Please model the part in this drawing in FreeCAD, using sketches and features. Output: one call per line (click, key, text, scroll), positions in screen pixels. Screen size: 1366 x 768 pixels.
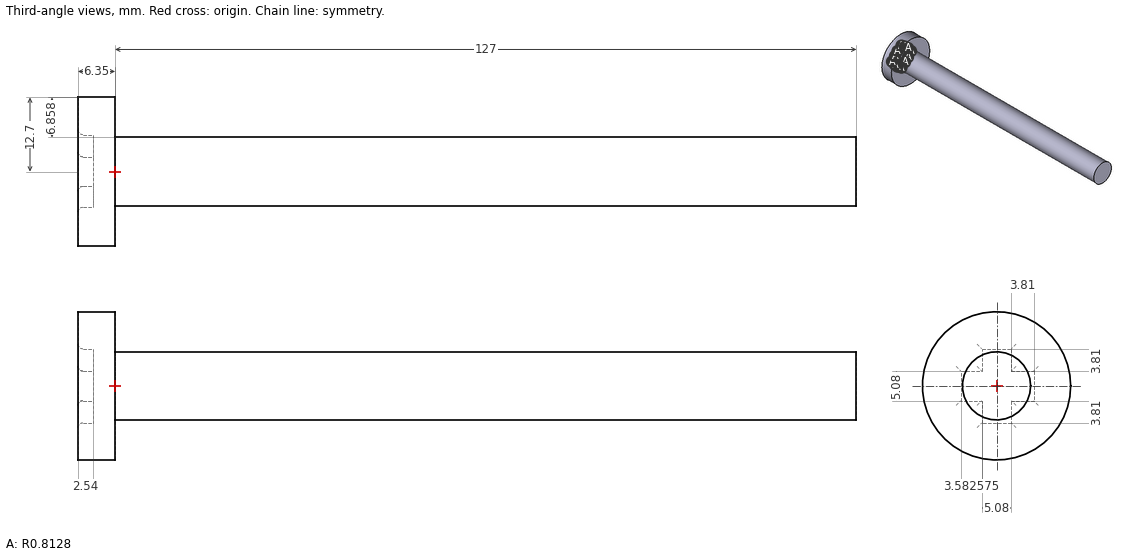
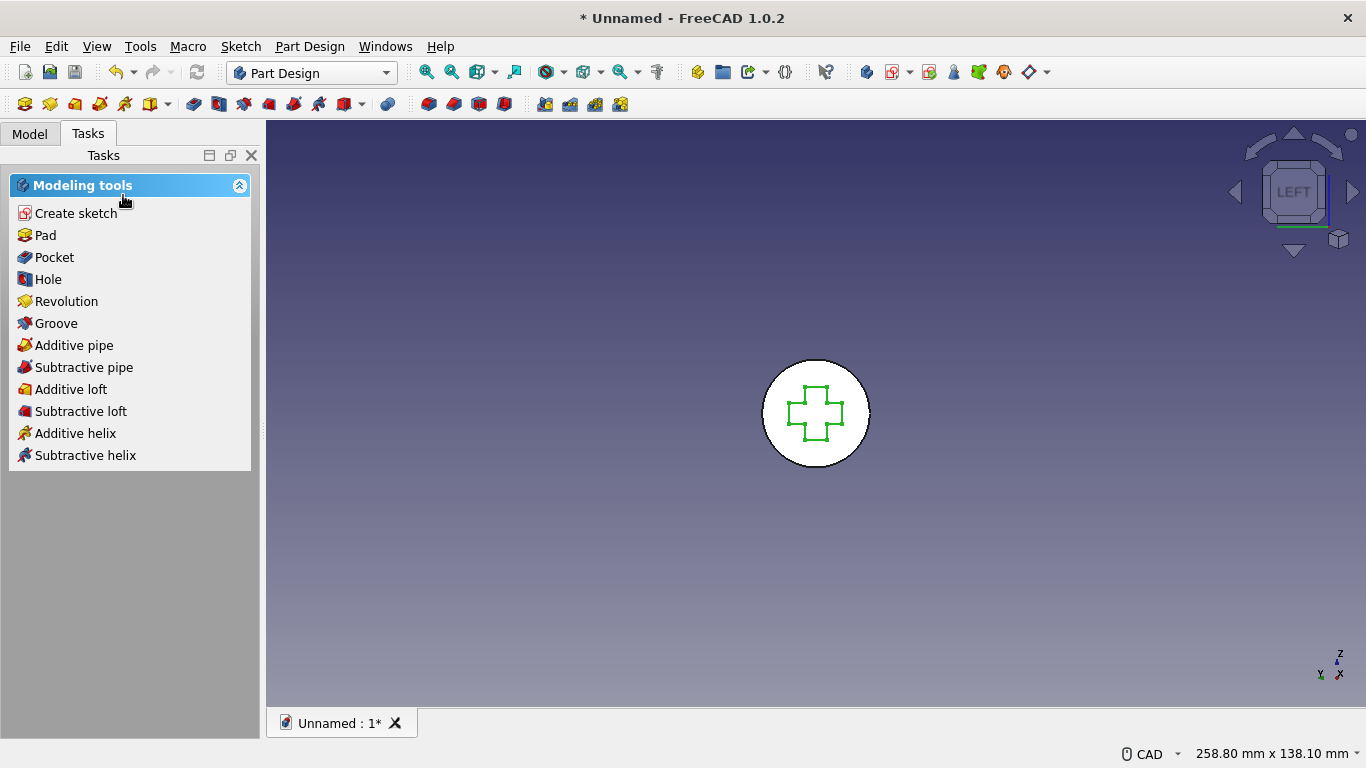
click(194, 104)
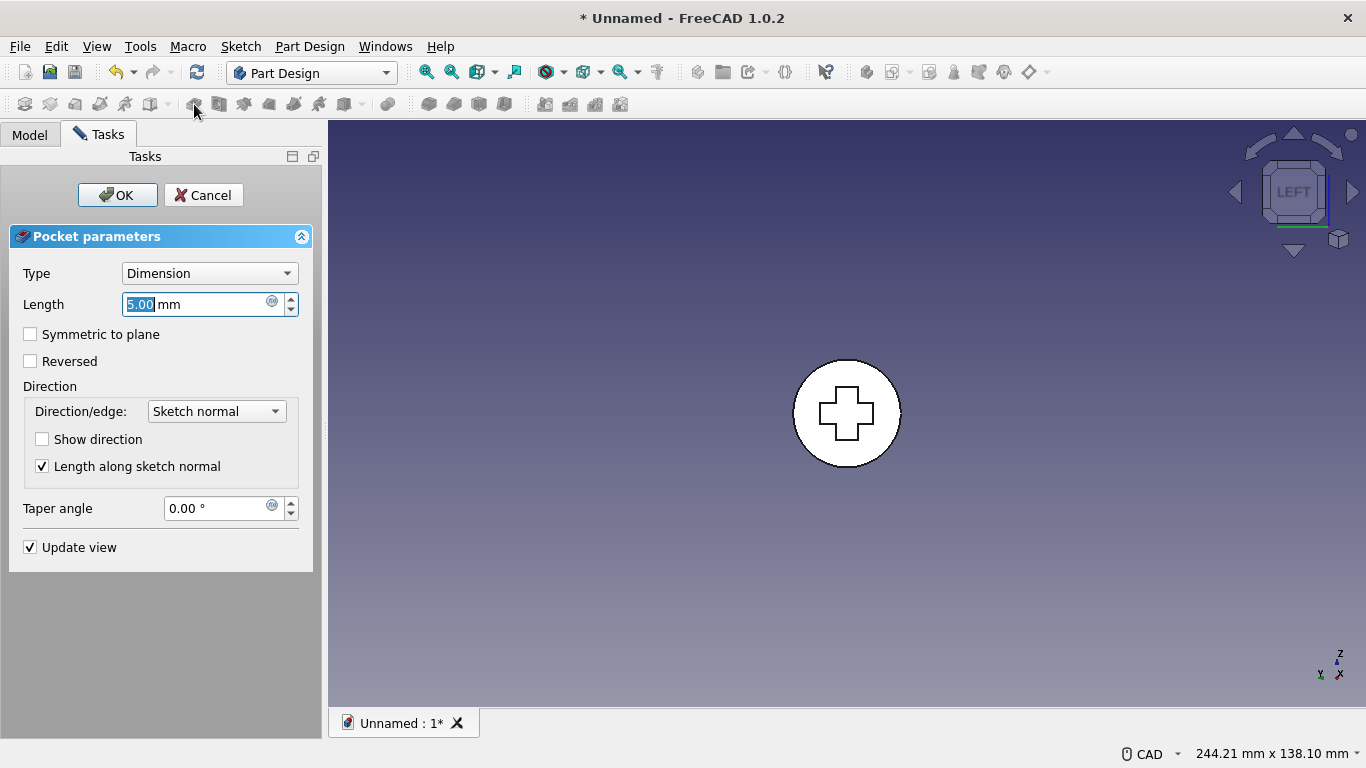
text(2.54)
key(Tab)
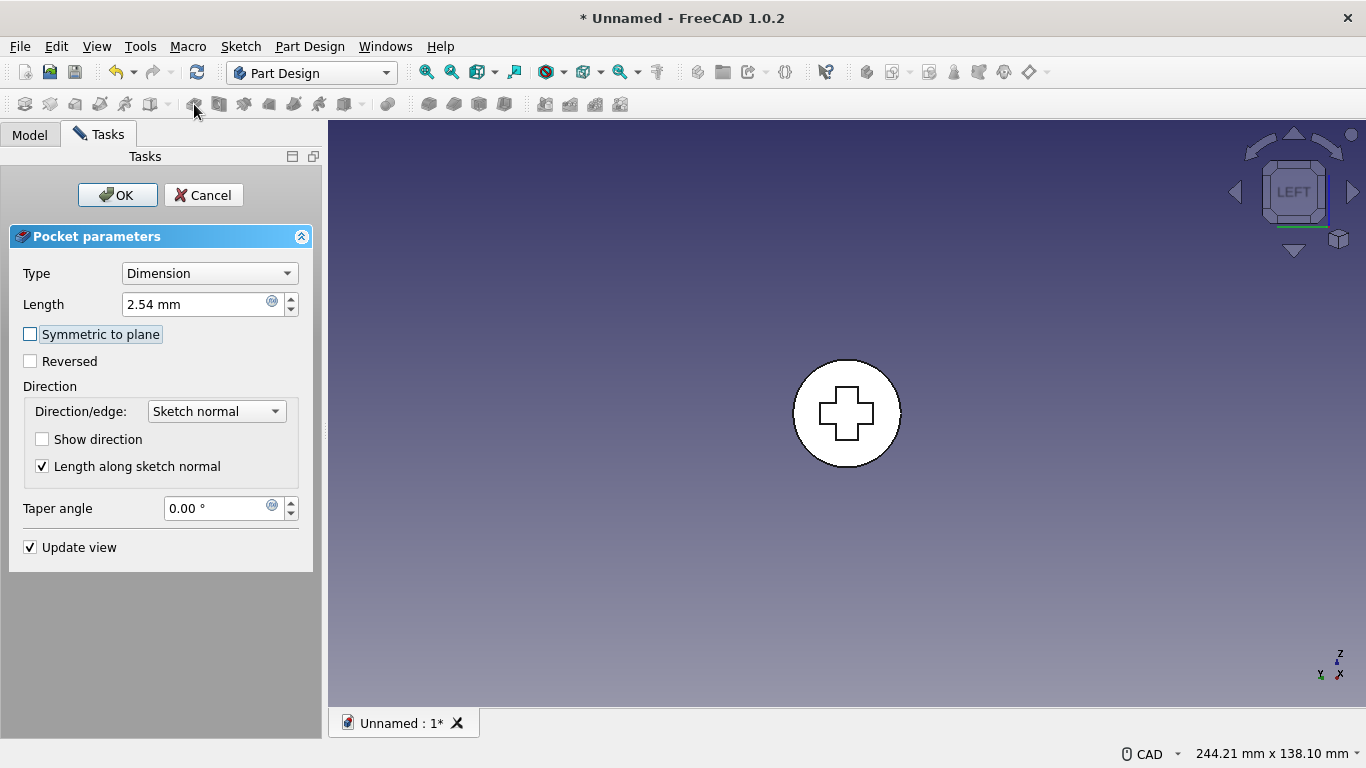
click(118, 195)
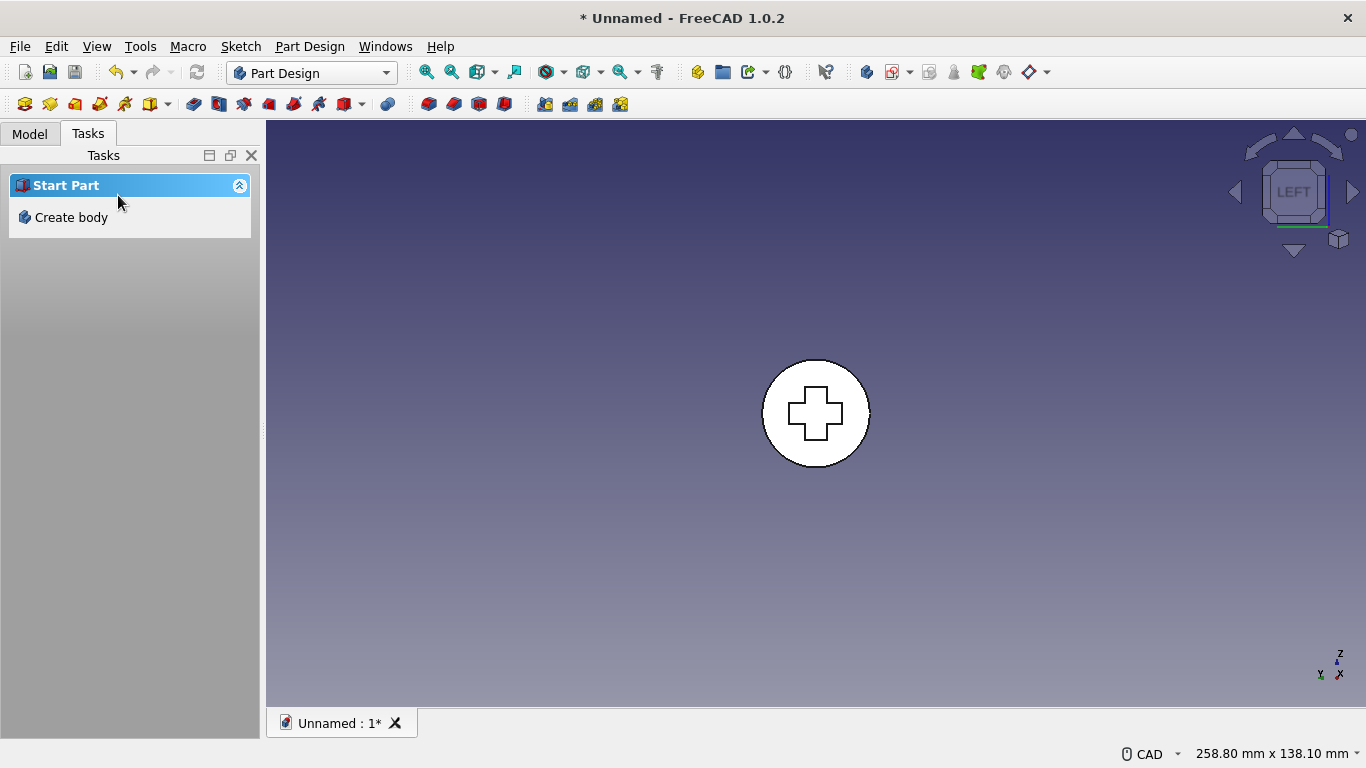
click(427, 72)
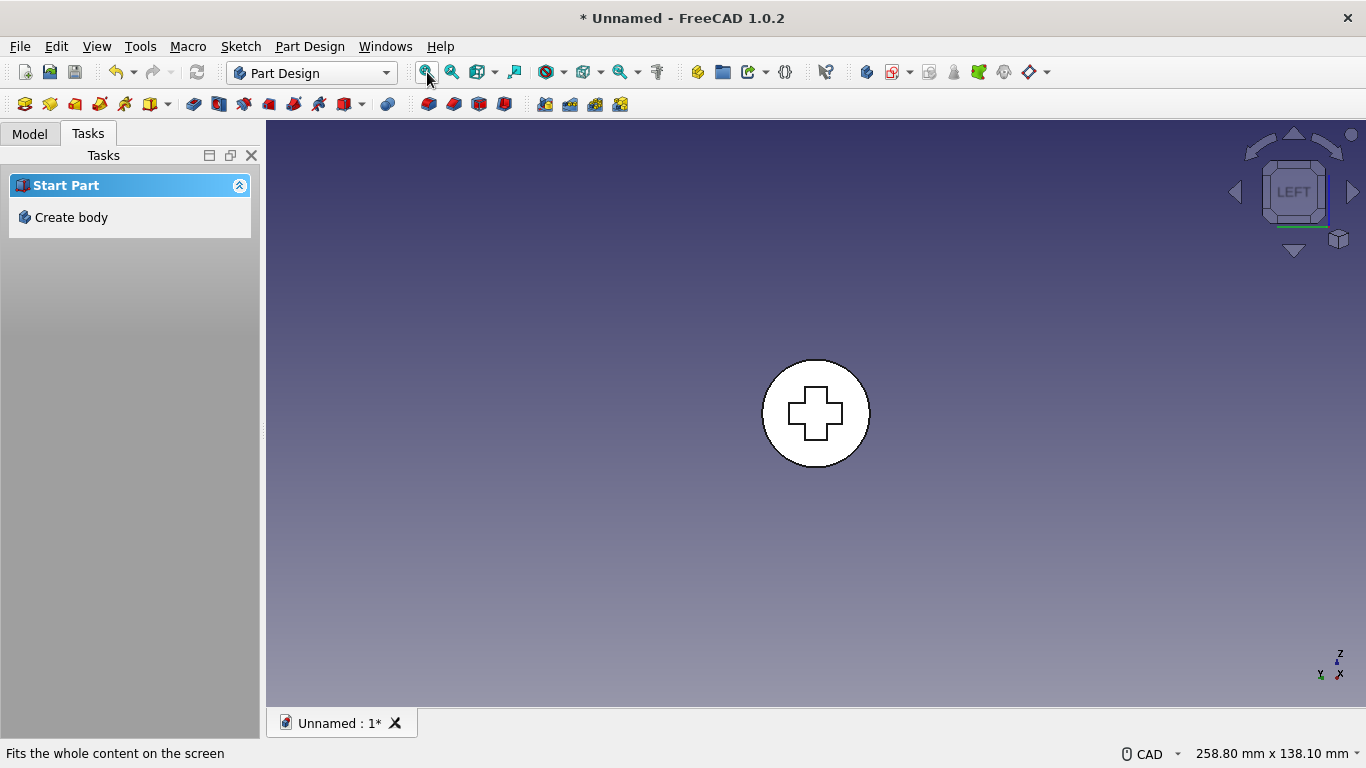
click(789, 412)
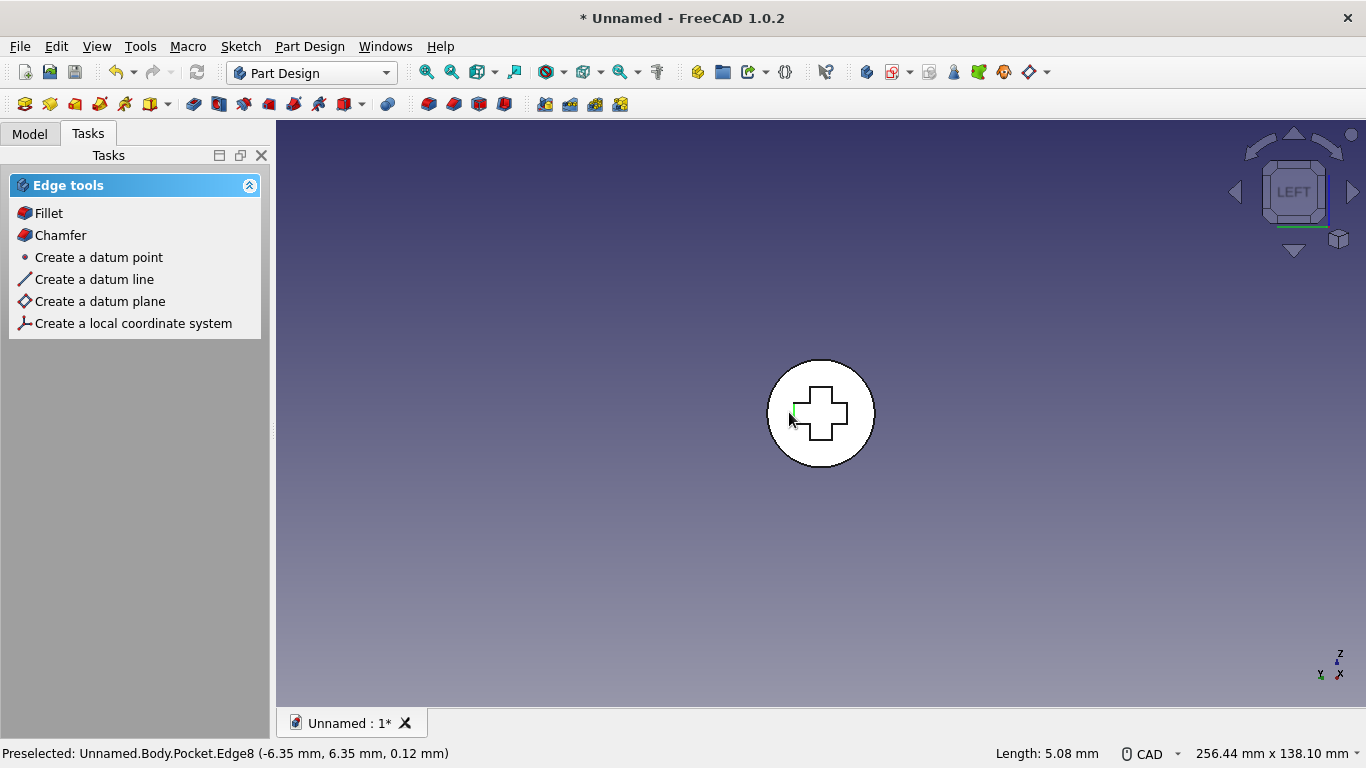
click(802, 423, ctrl)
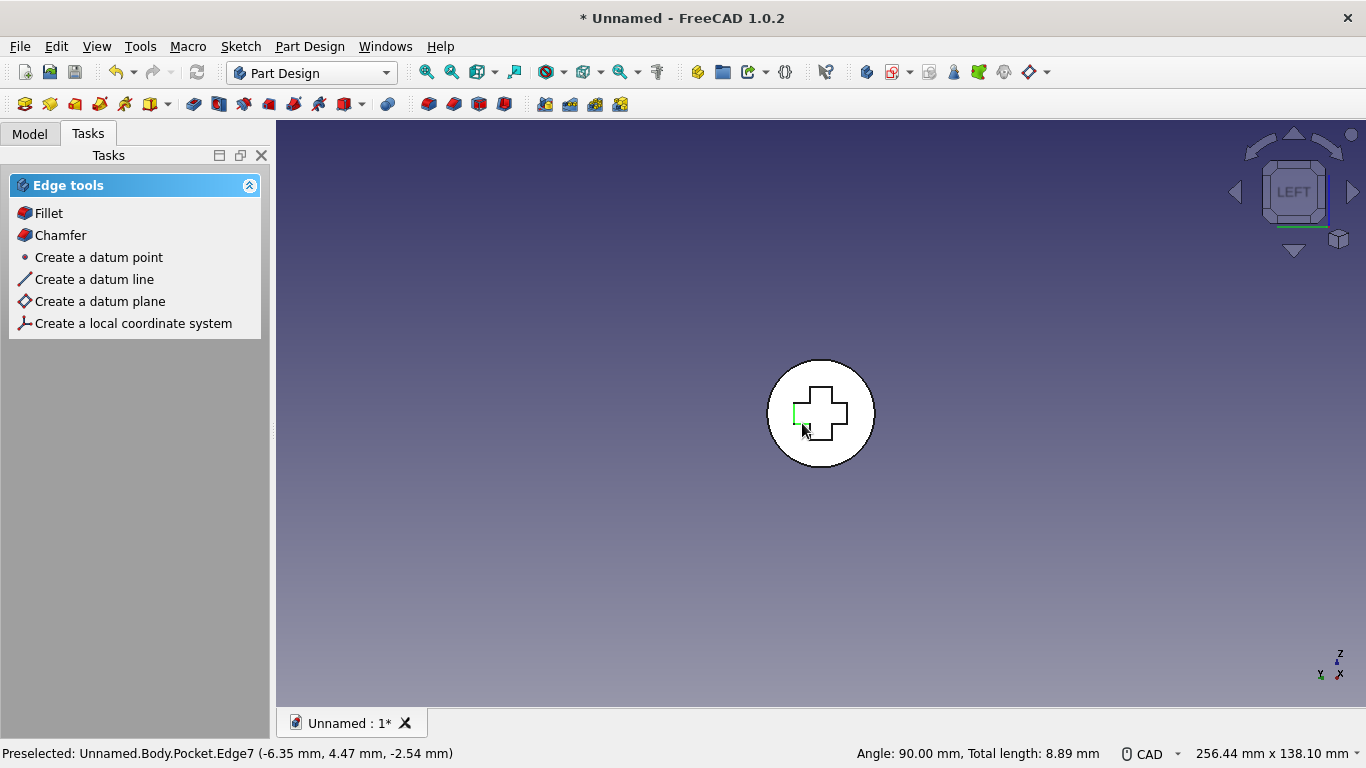
click(810, 431, ctrl)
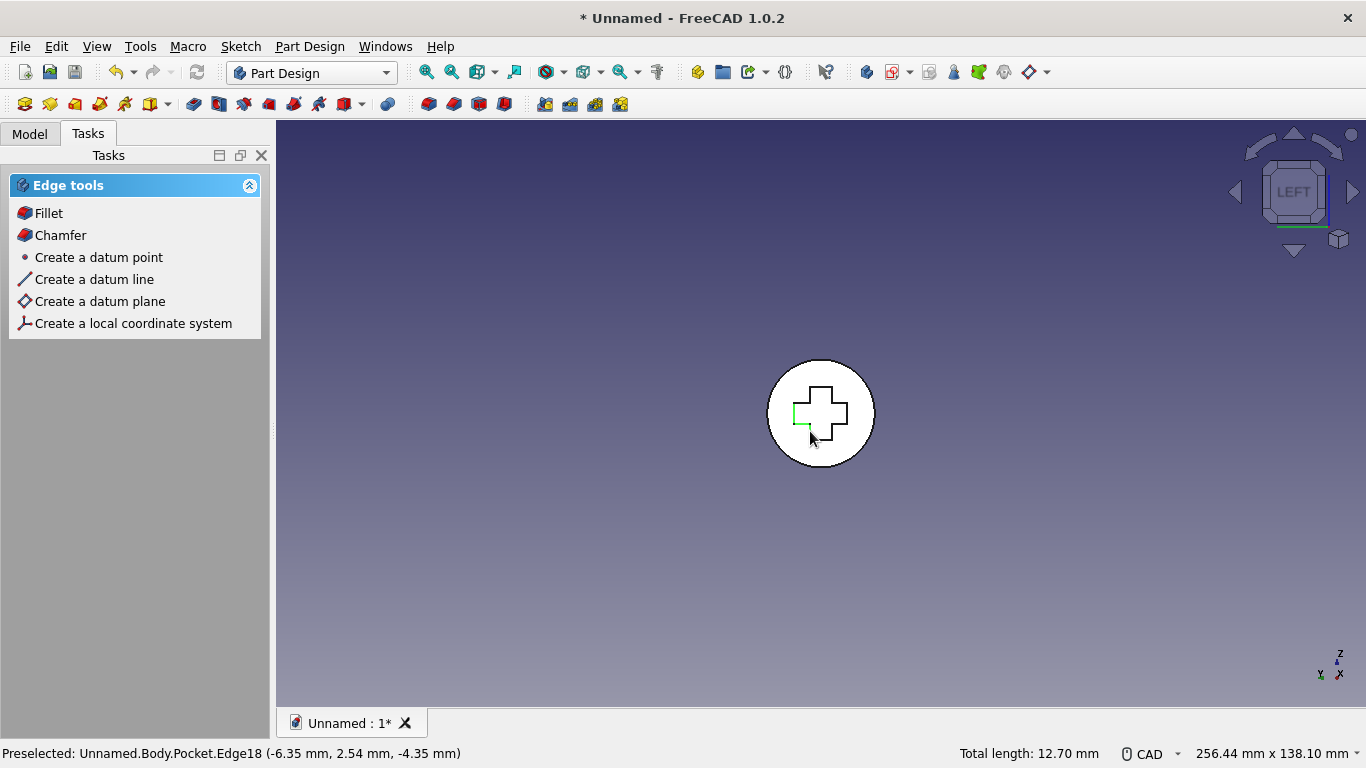
click(821, 439, ctrl)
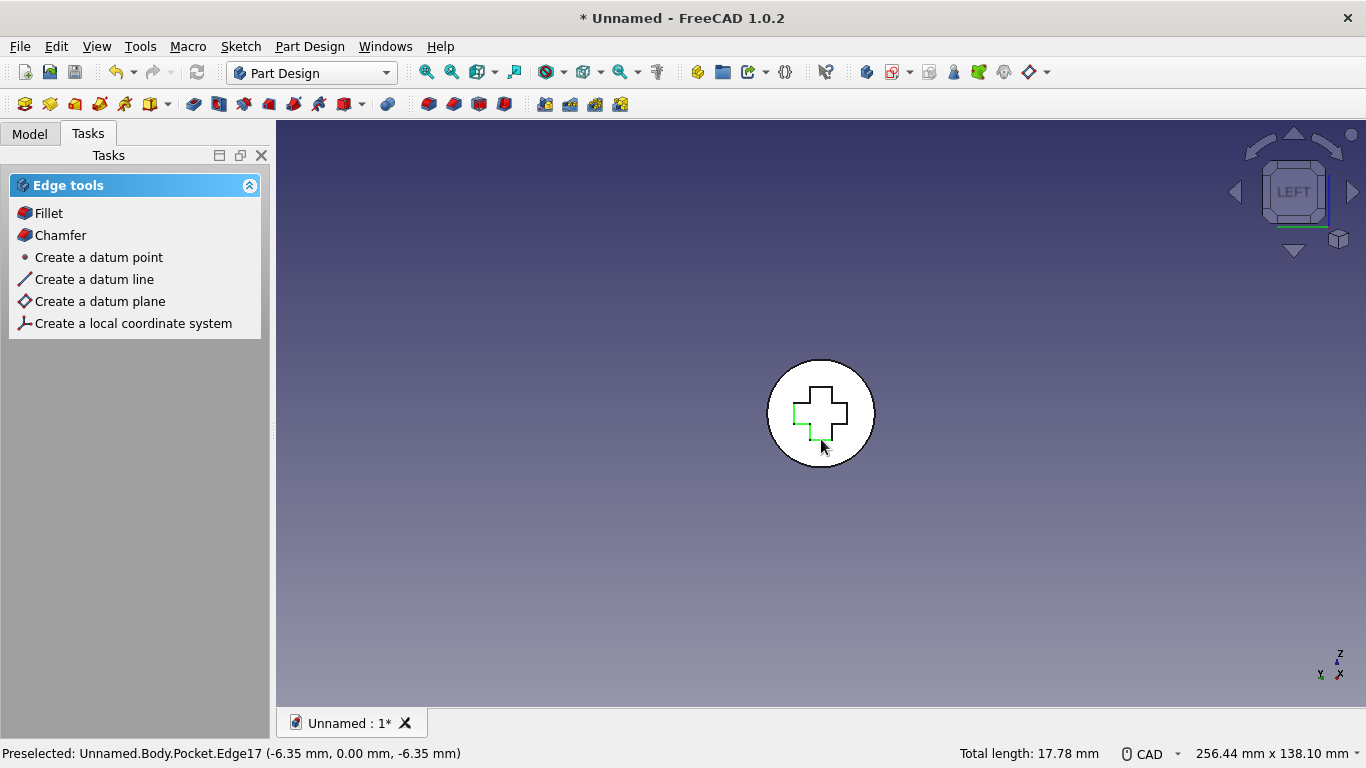
click(832, 431, ctrl)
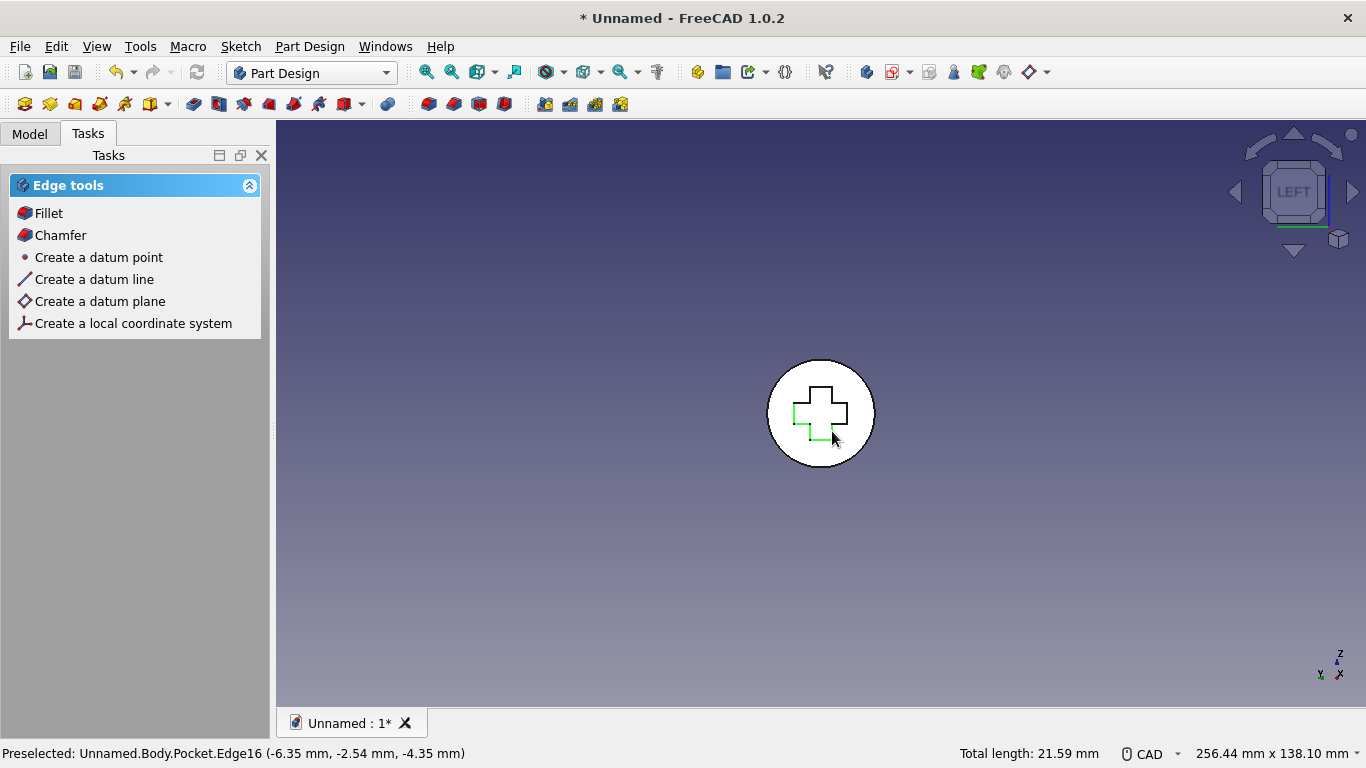
click(839, 423, ctrl)